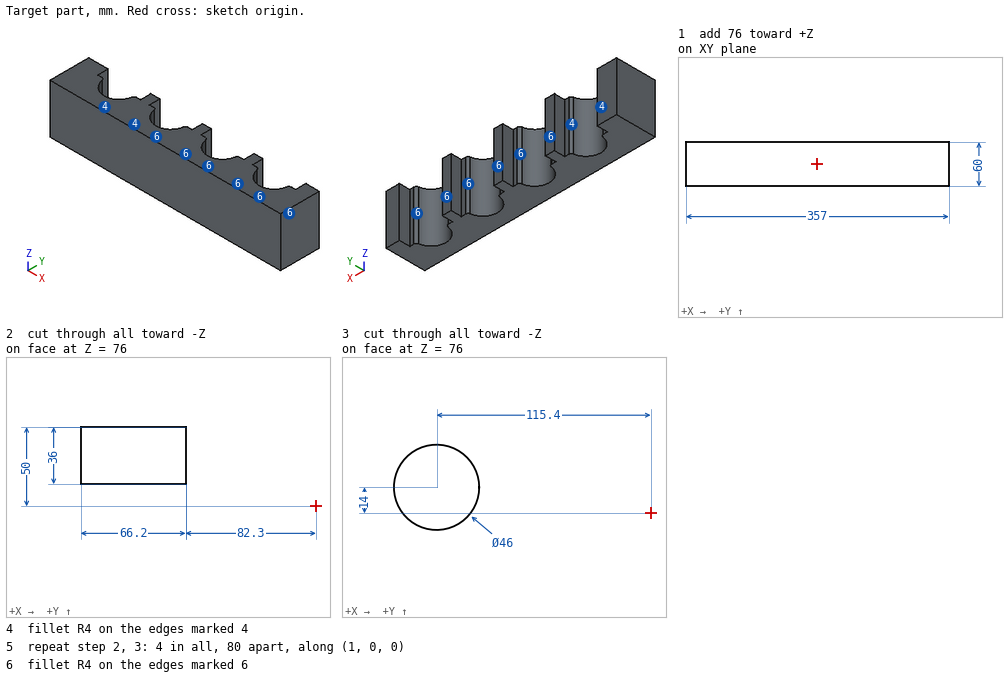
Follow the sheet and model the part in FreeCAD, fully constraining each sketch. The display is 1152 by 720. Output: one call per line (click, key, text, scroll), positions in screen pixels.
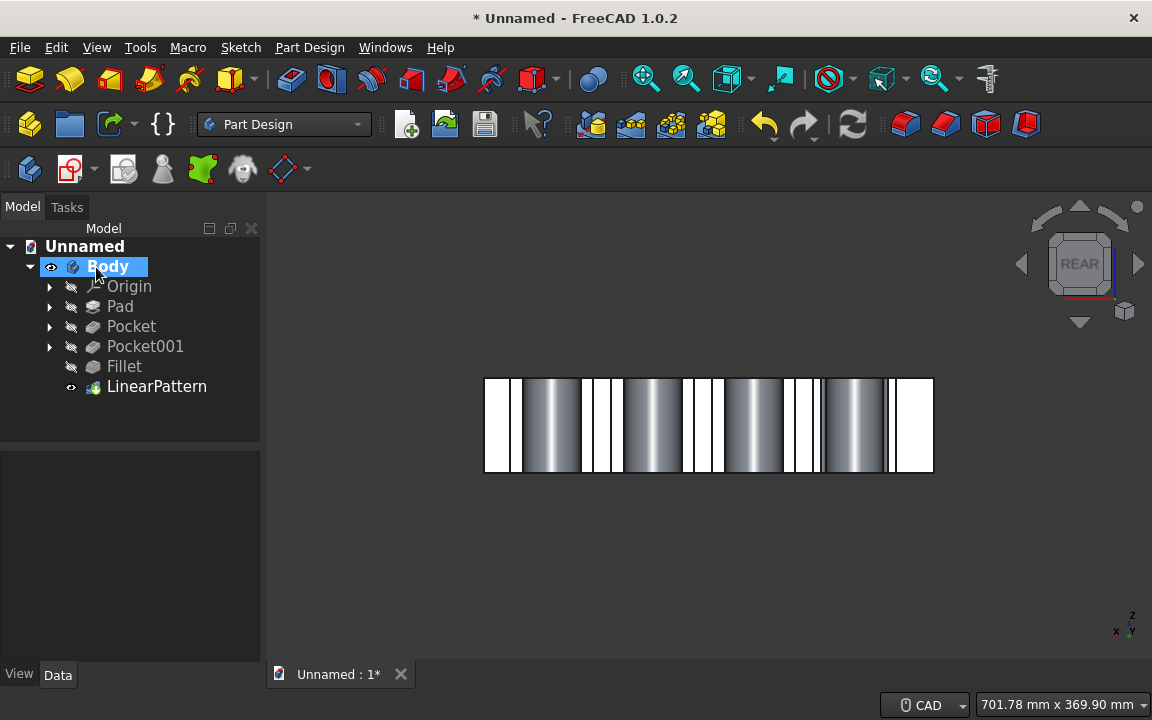
click(783, 424)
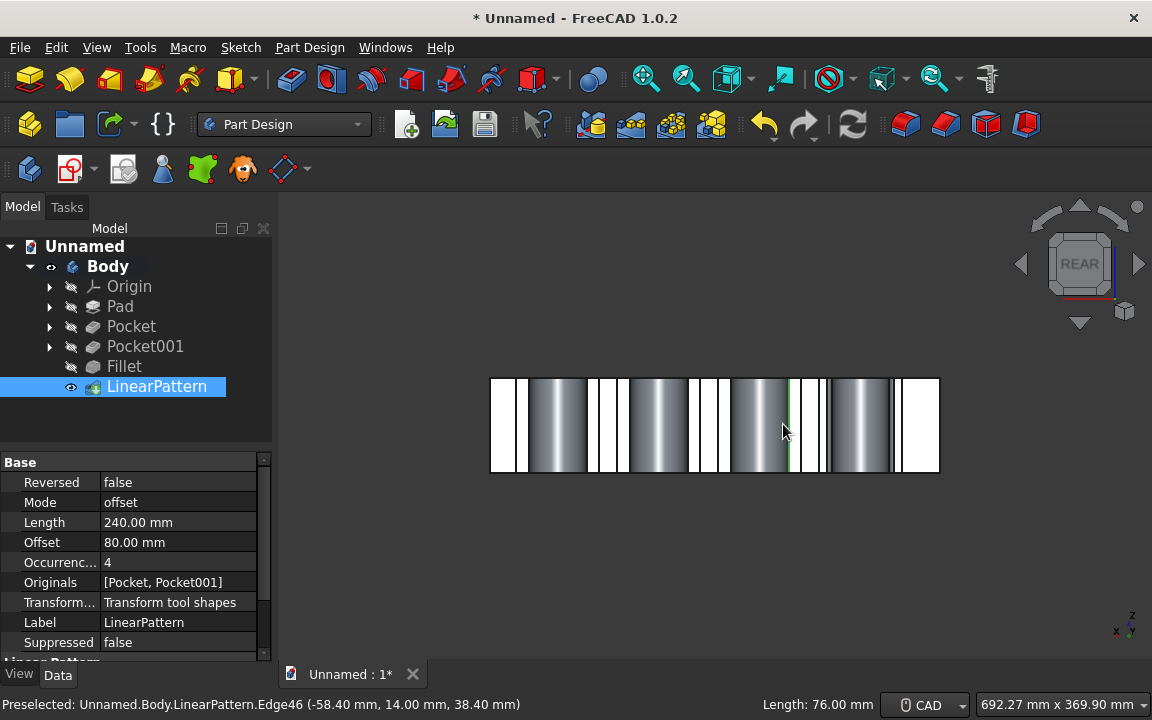
click(731, 424, ctrl)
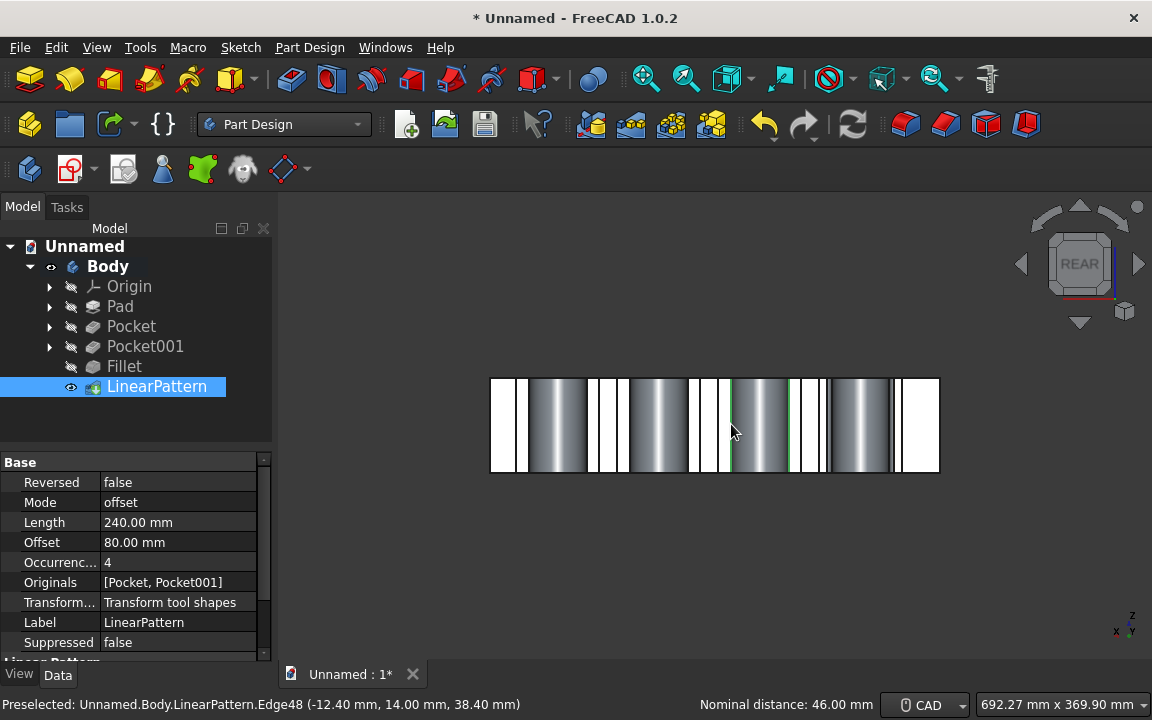
click(688, 424, ctrl)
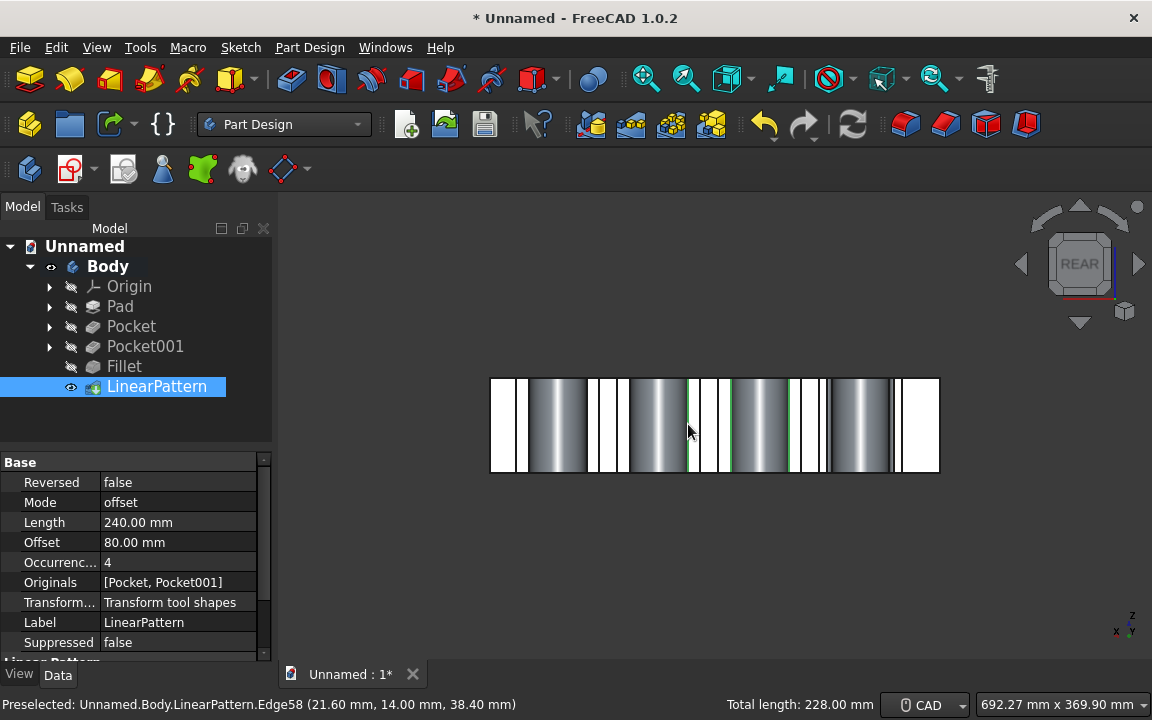
click(630, 424, ctrl)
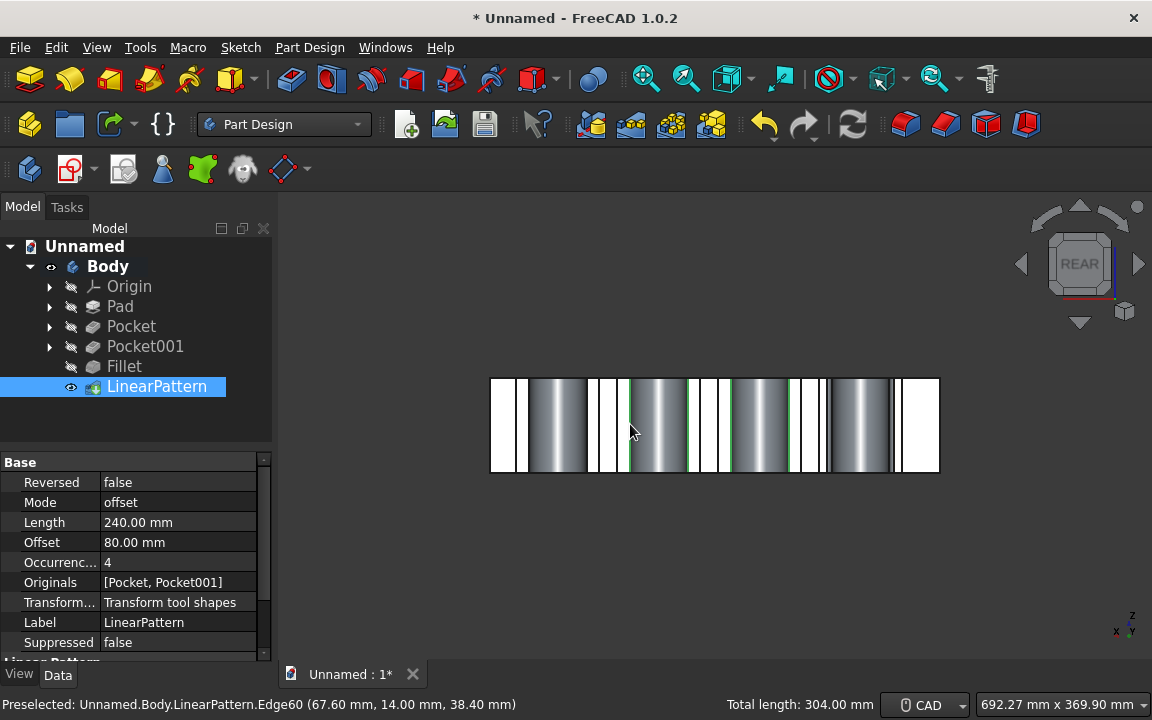
click(587, 424, ctrl)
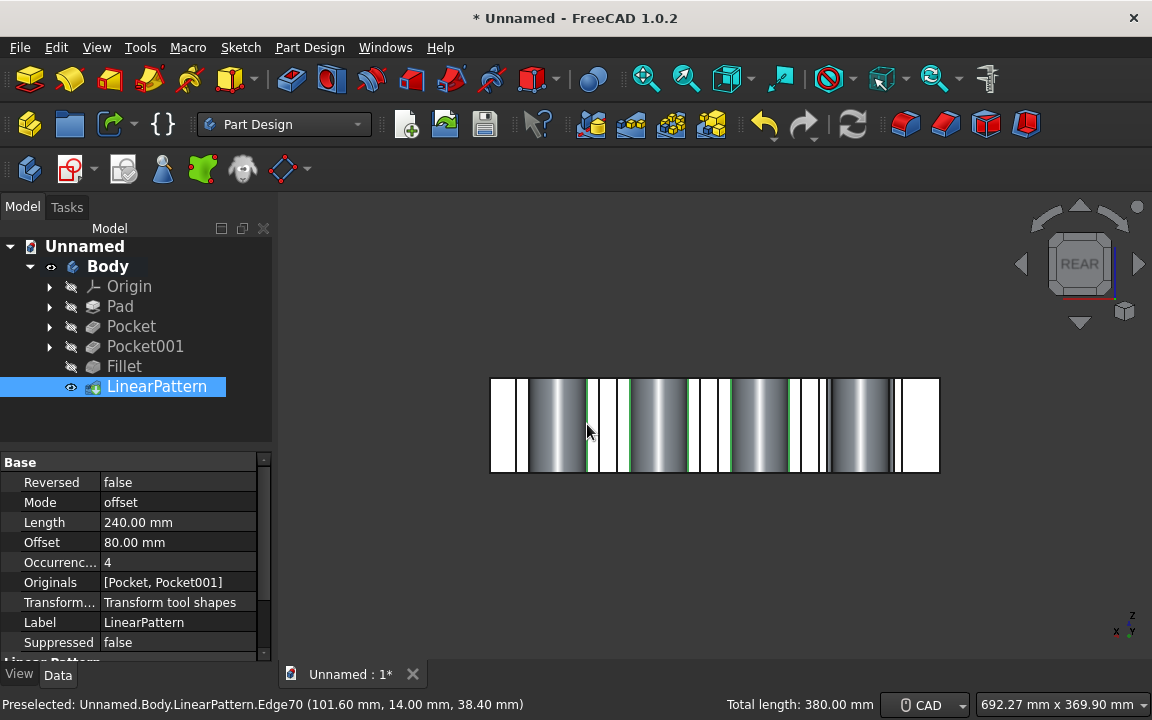
click(529, 424, ctrl)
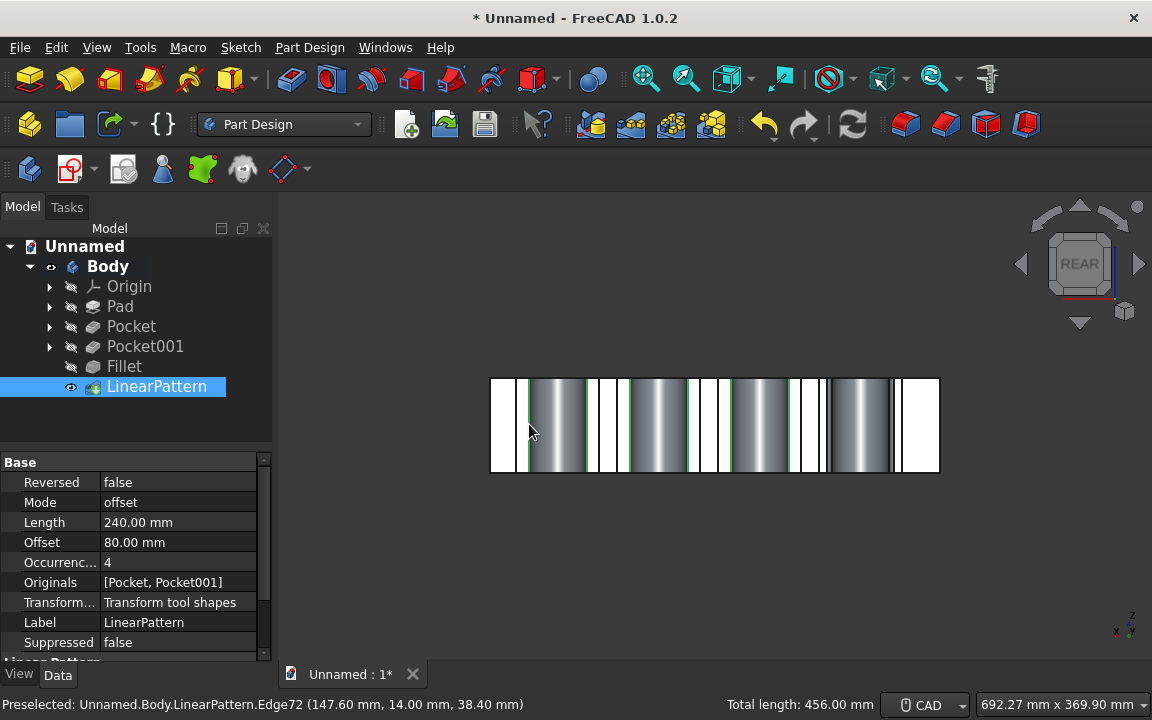
click(906, 124)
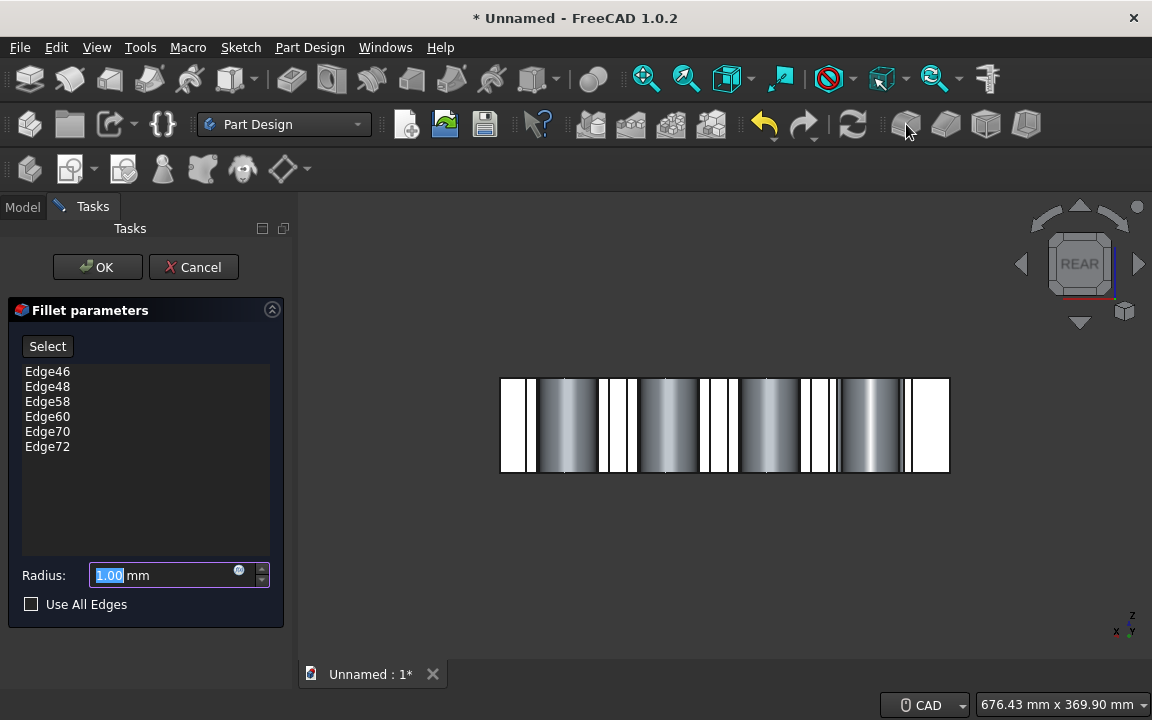
text(4)
key(Tab)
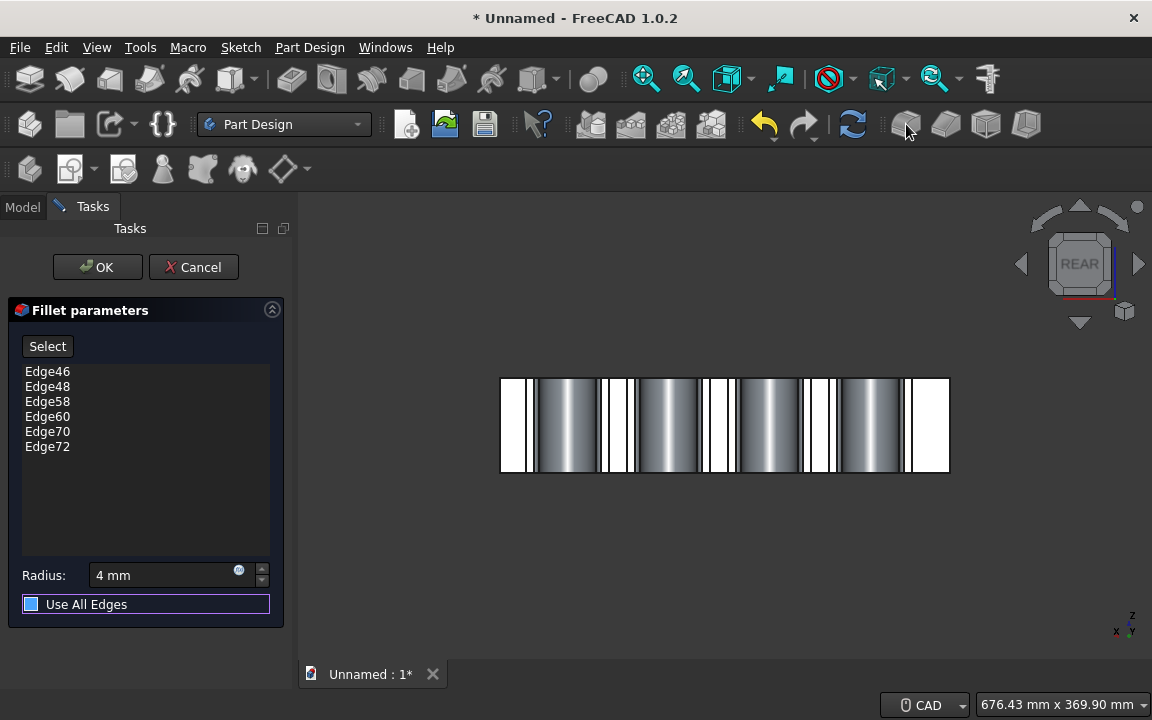
click(98, 267)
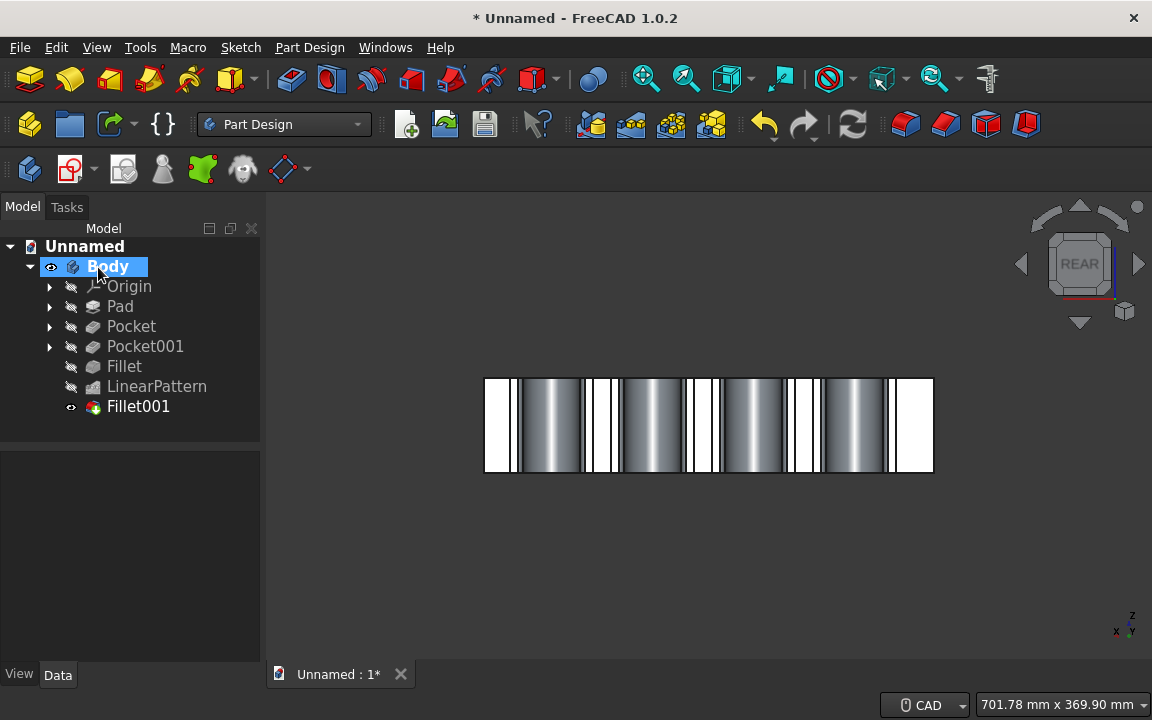
key(0)